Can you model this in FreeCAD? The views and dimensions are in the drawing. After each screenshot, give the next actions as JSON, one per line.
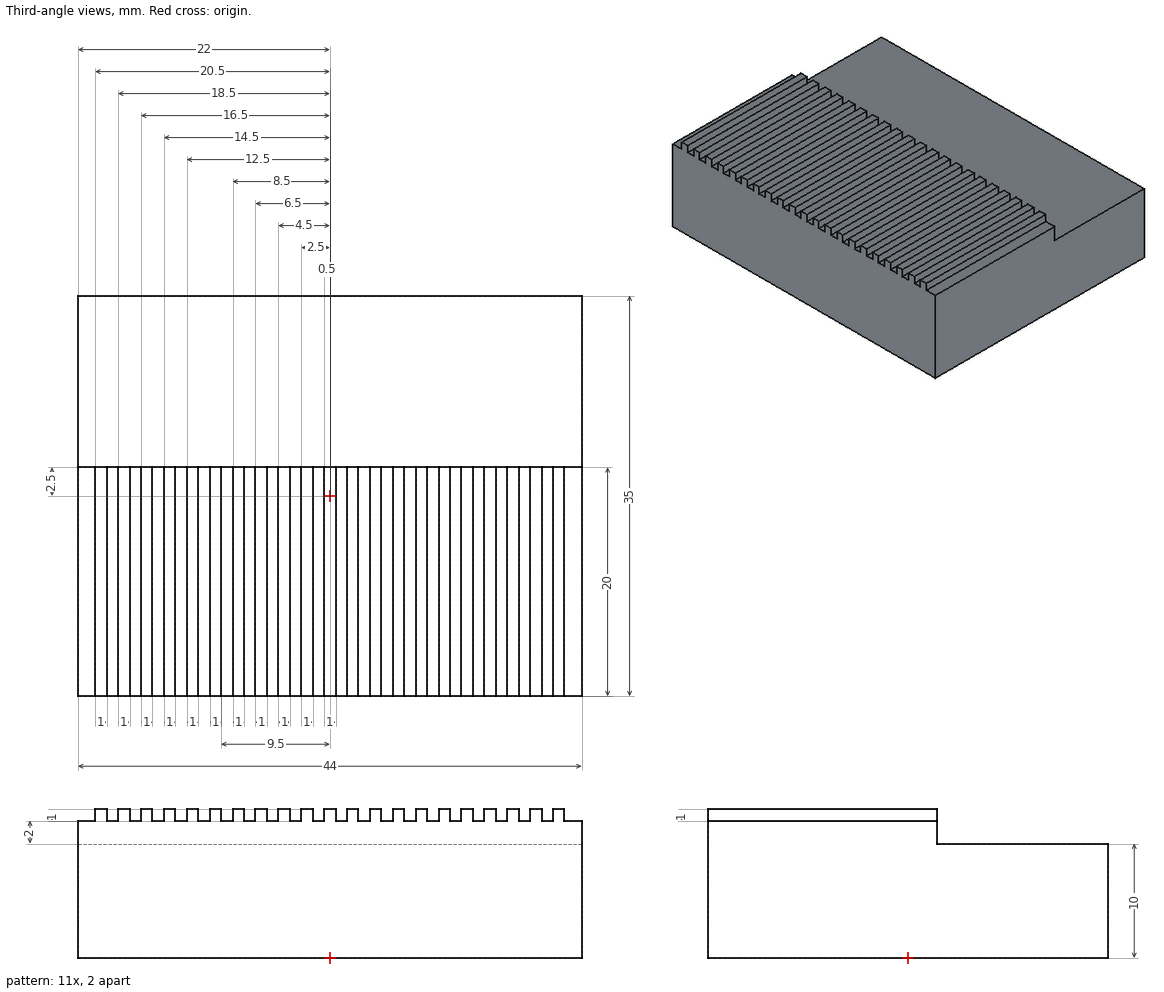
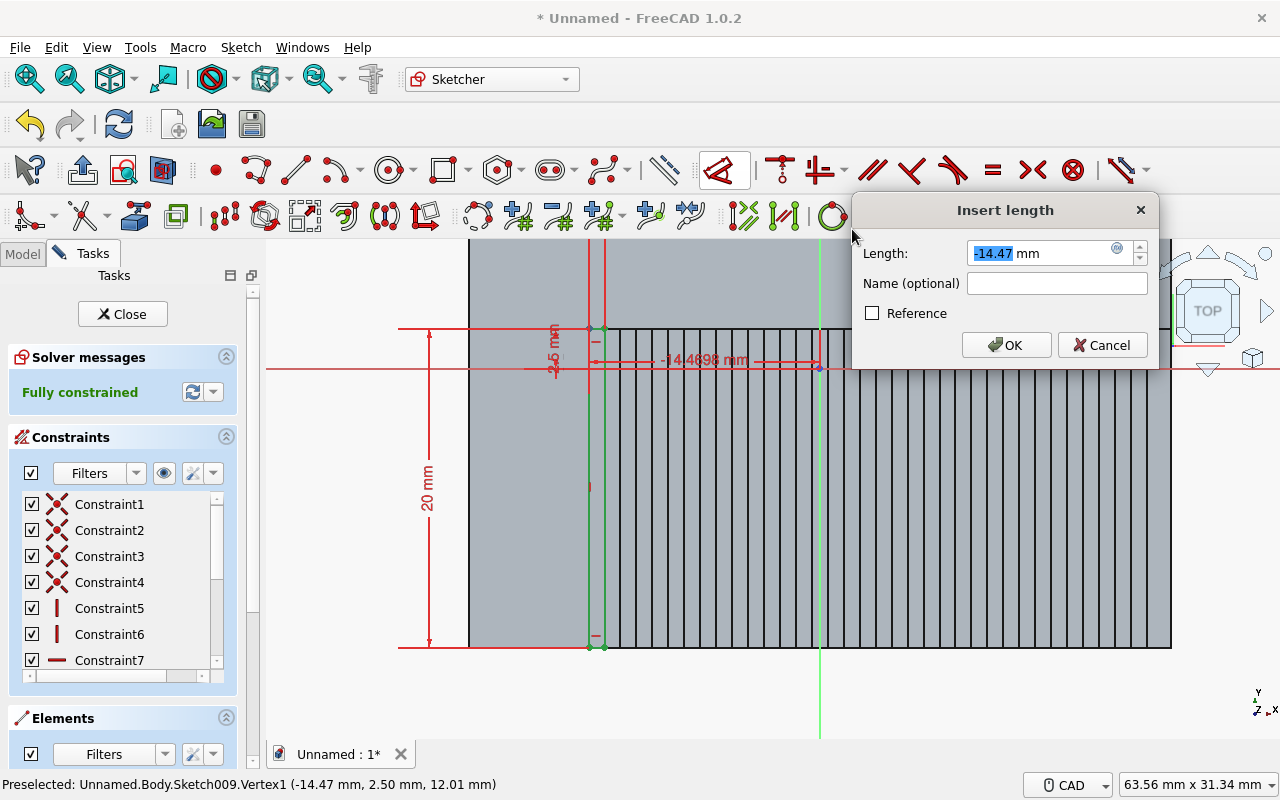
{"action": "type", "text": "-14.5"}
{"action": "key", "text": "Return"}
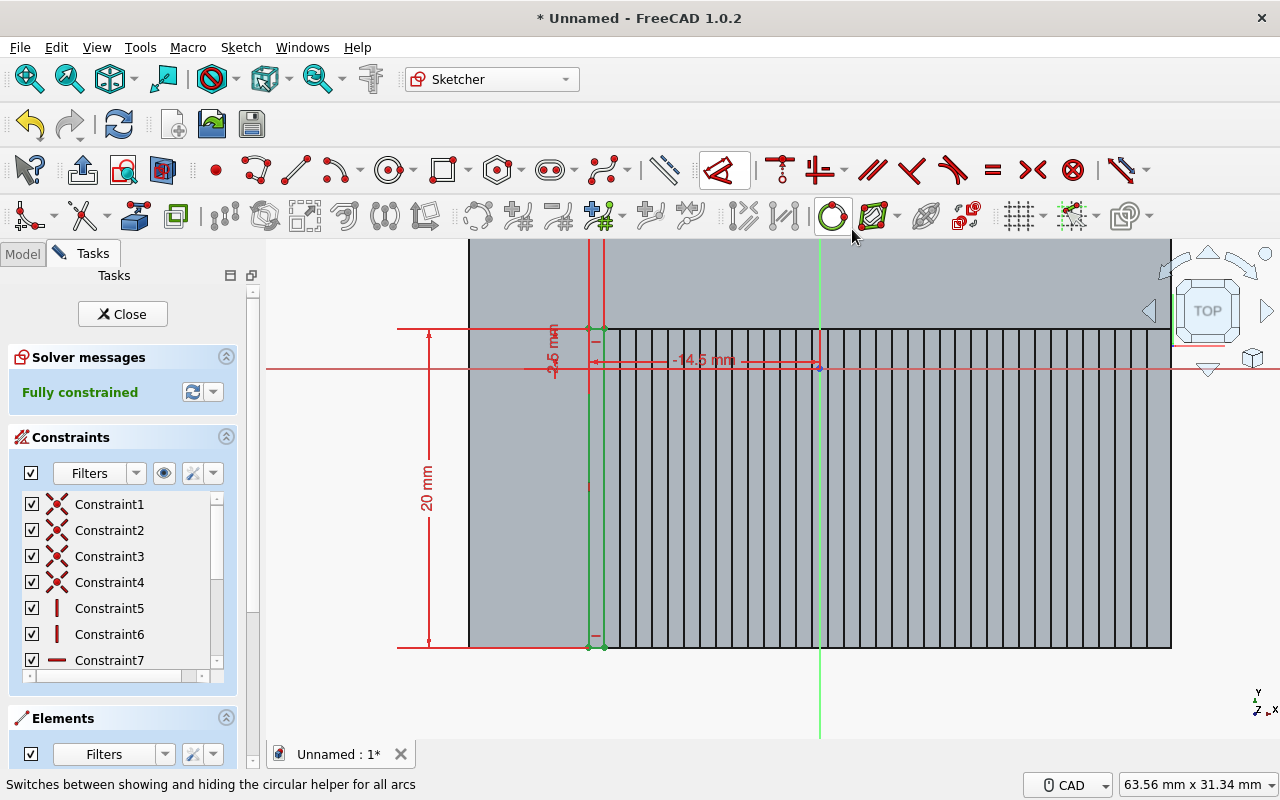
{"action": "left_click", "coordinate": [123, 314]}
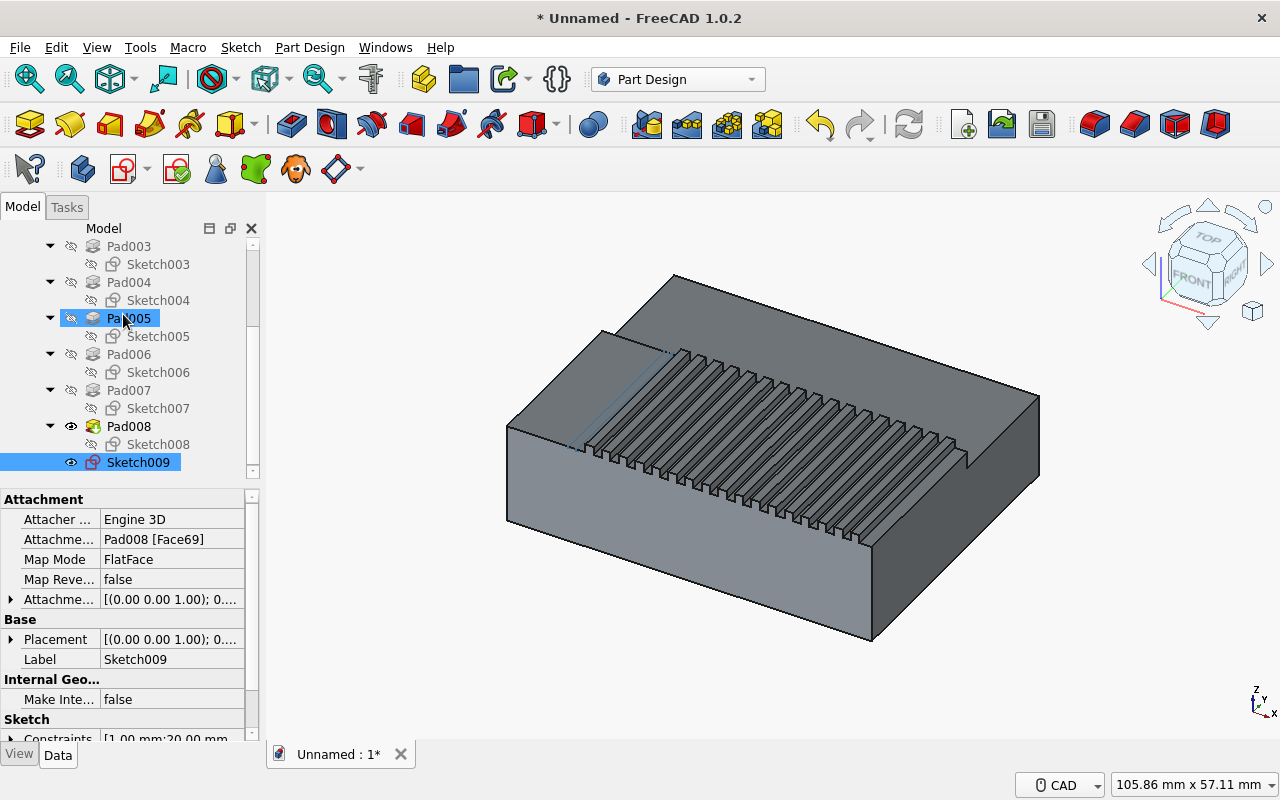
{"action": "left_click", "coordinate": [30, 124]}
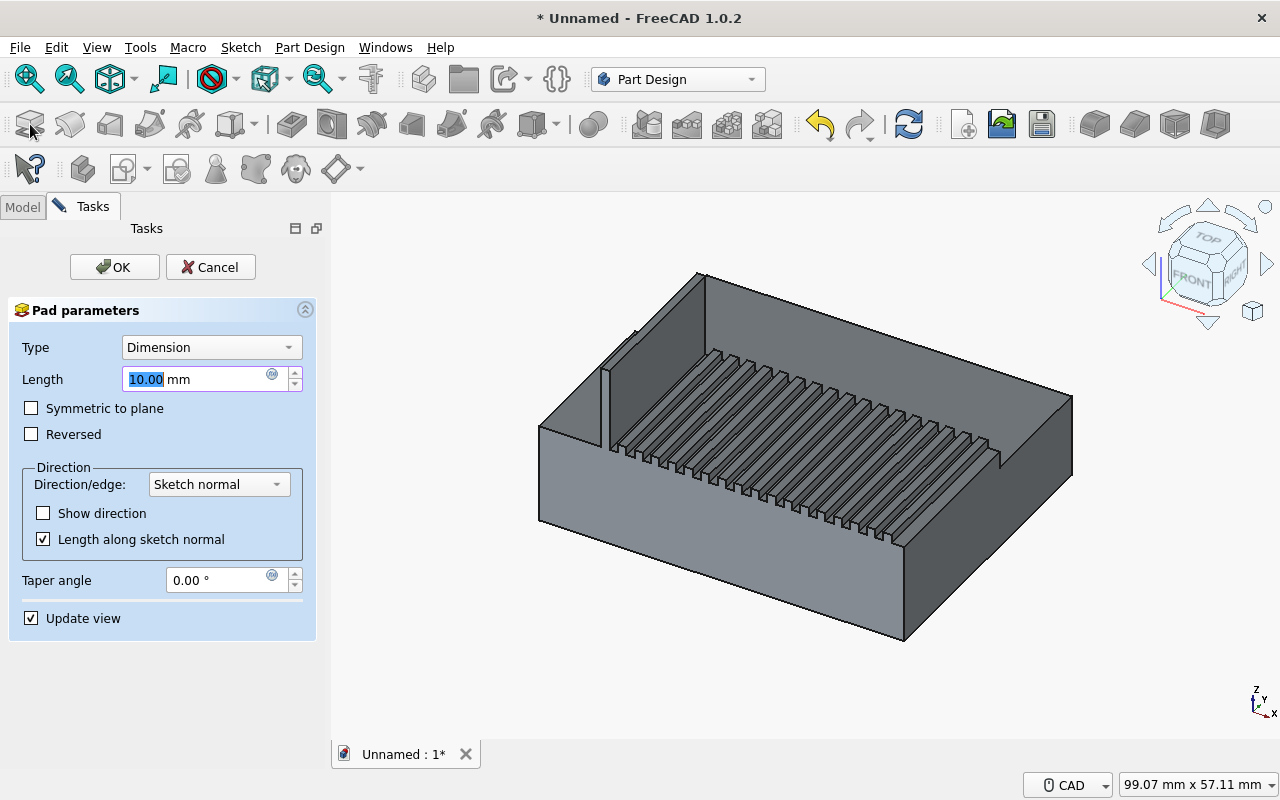
{"action": "type", "text": "1"}
{"action": "key", "text": "Tab"}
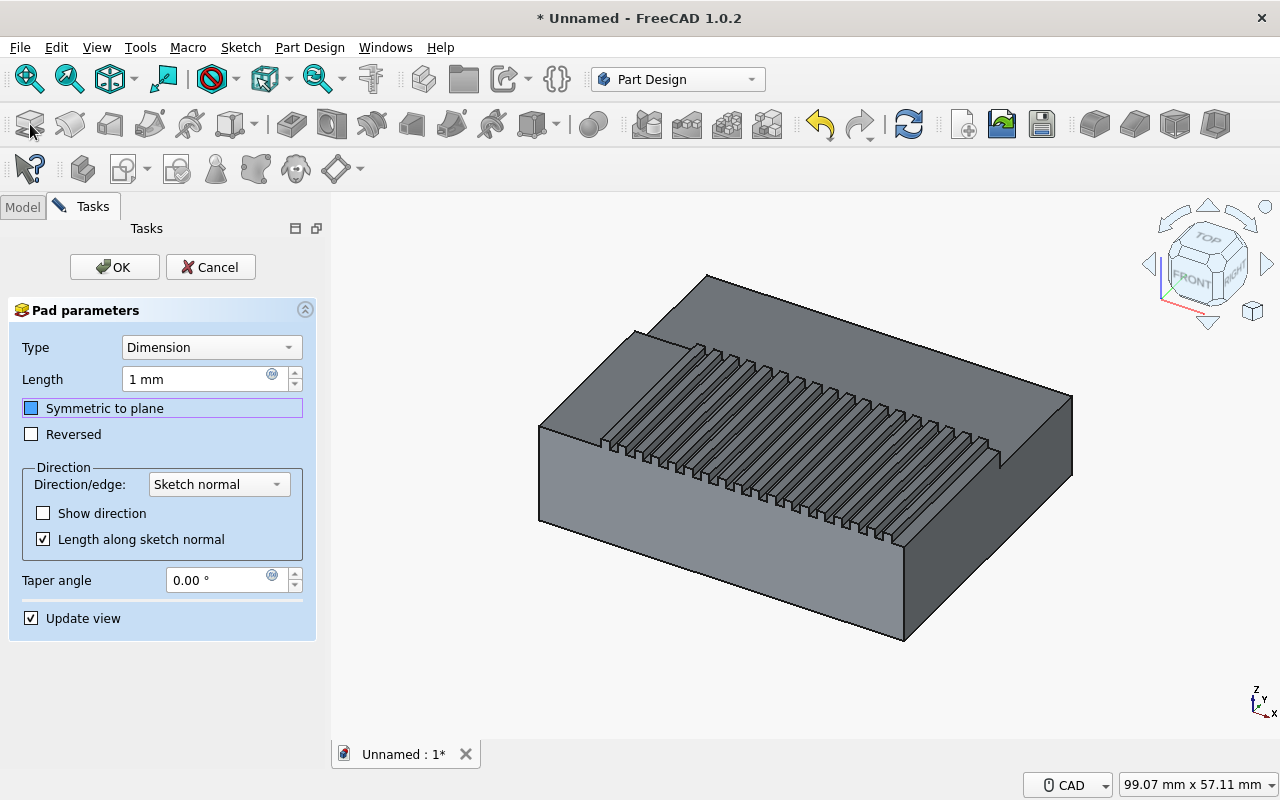
{"action": "left_click", "coordinate": [115, 267]}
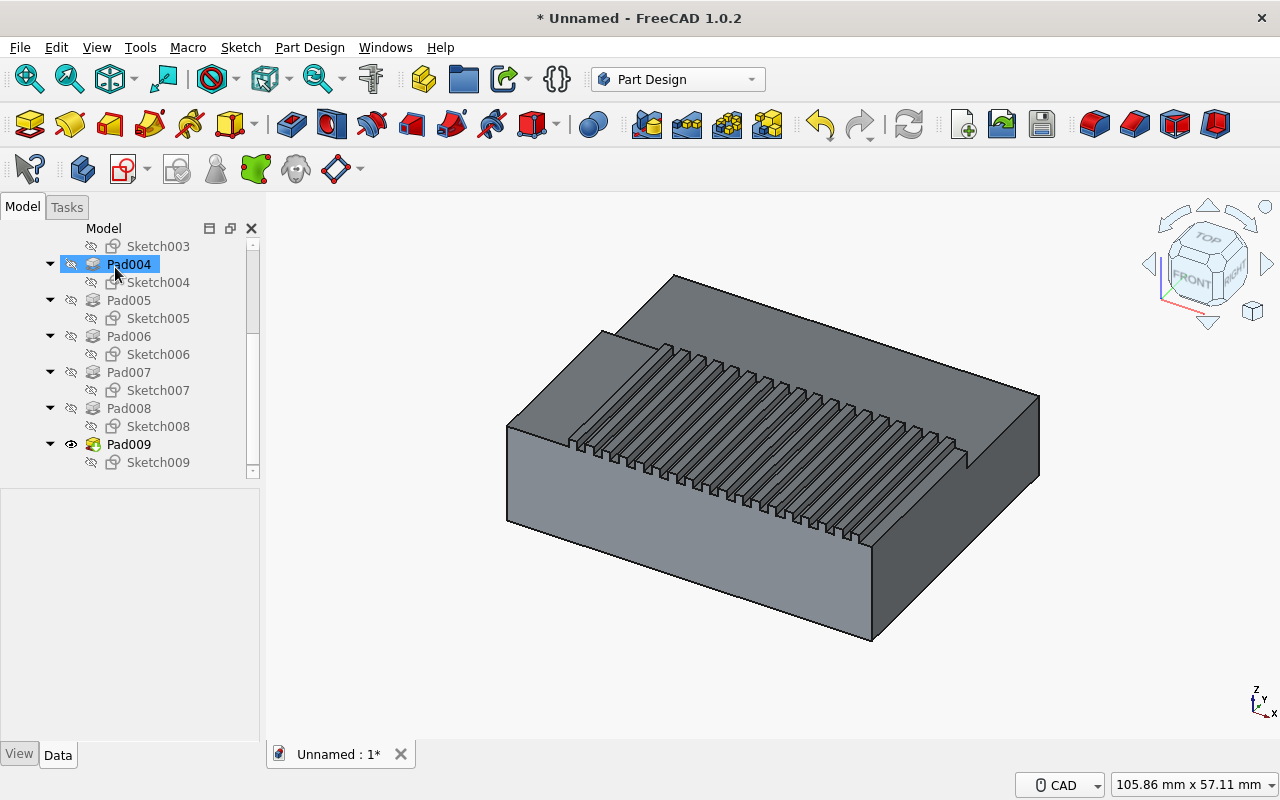
{"action": "left_click", "coordinate": [613, 361]}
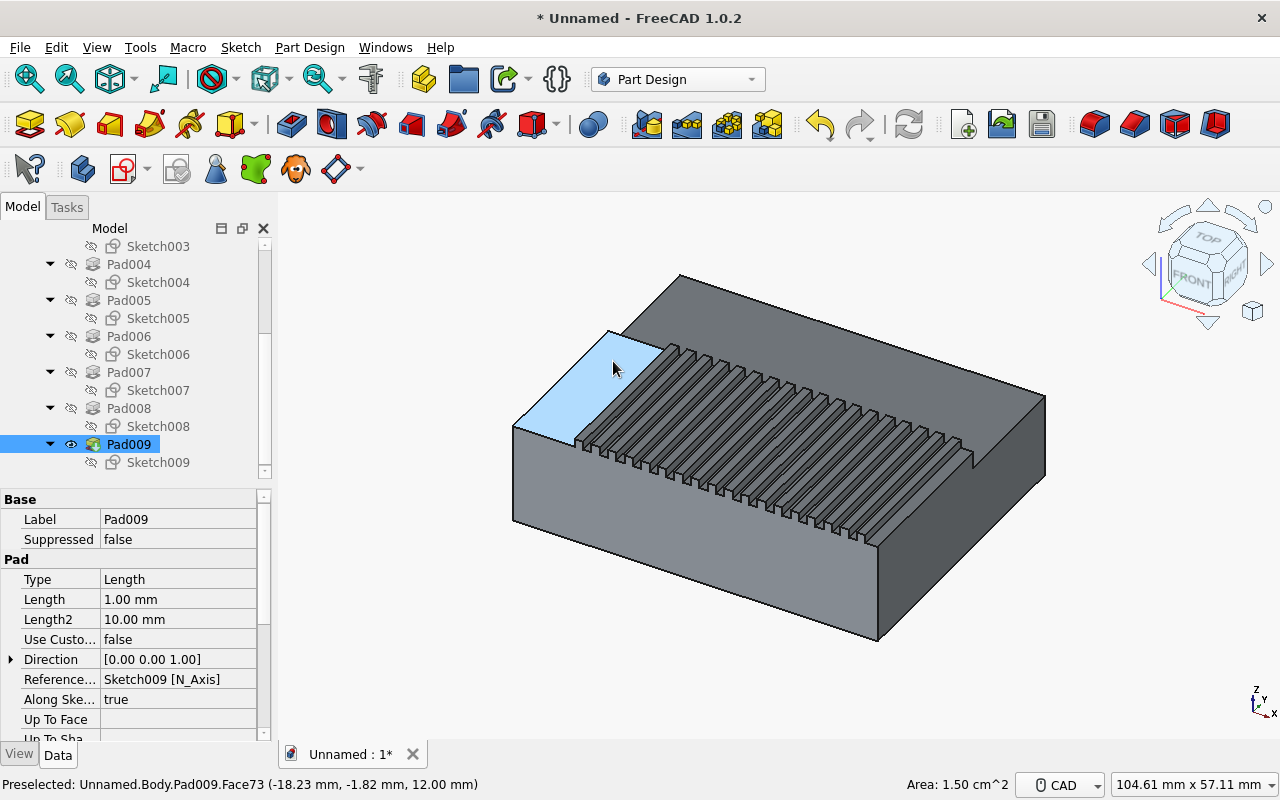
{"action": "left_click", "coordinate": [124, 170]}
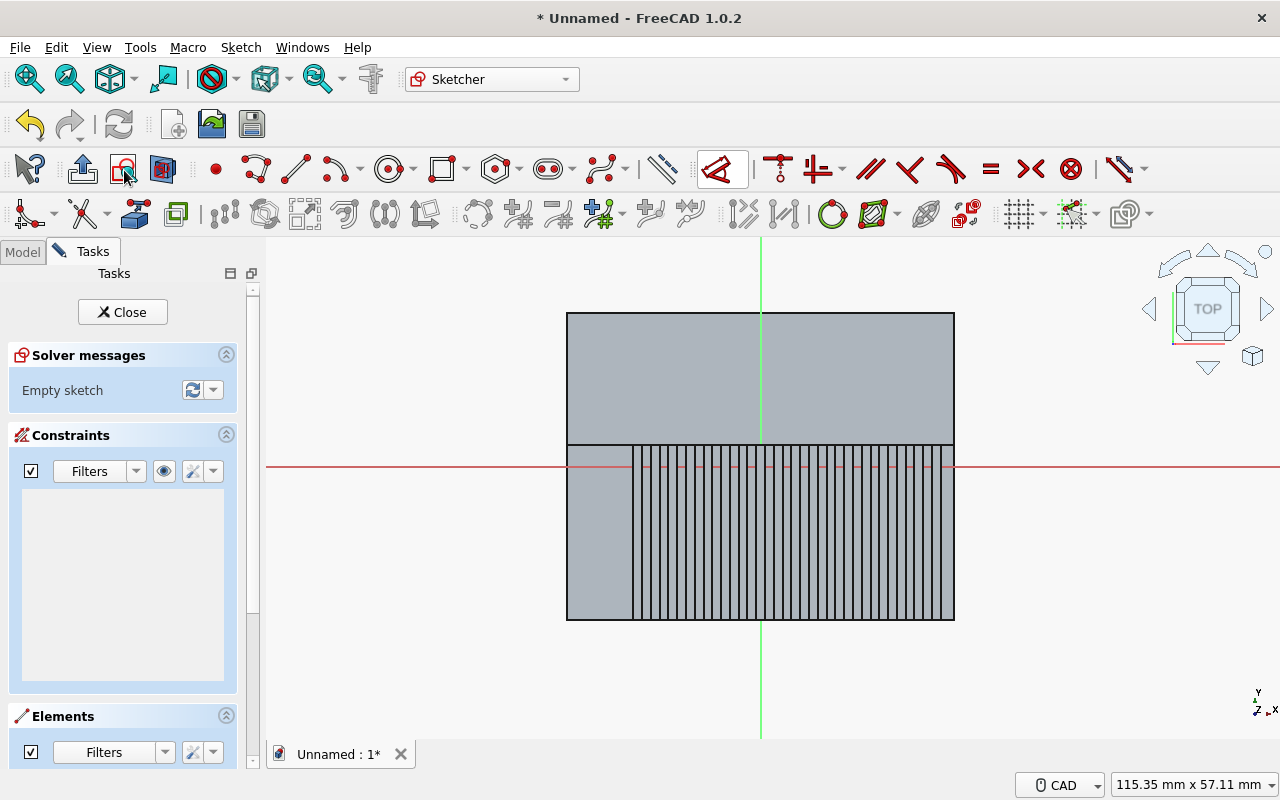
{"action": "scroll", "coordinate": [668, 587], "scroll_direction": "up", "scroll_amount": 3}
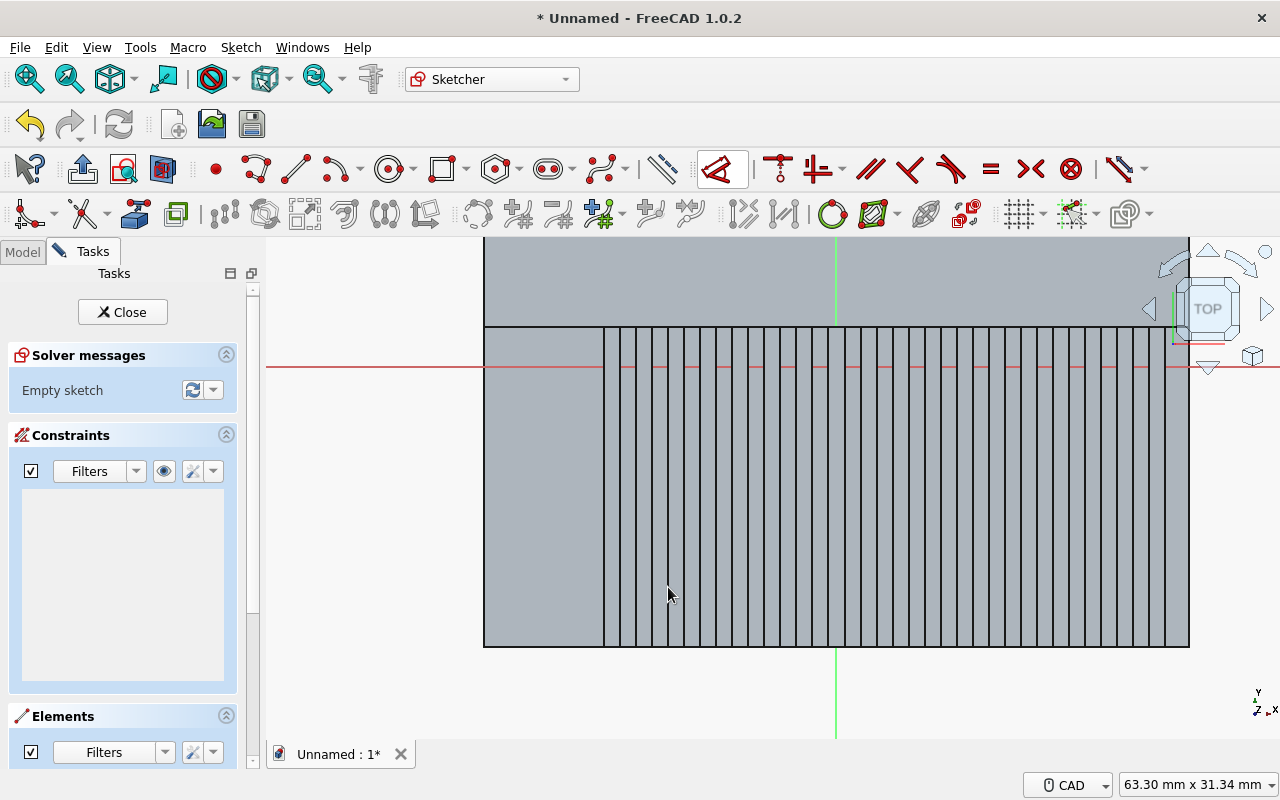
{"action": "left_click", "coordinate": [442, 170]}